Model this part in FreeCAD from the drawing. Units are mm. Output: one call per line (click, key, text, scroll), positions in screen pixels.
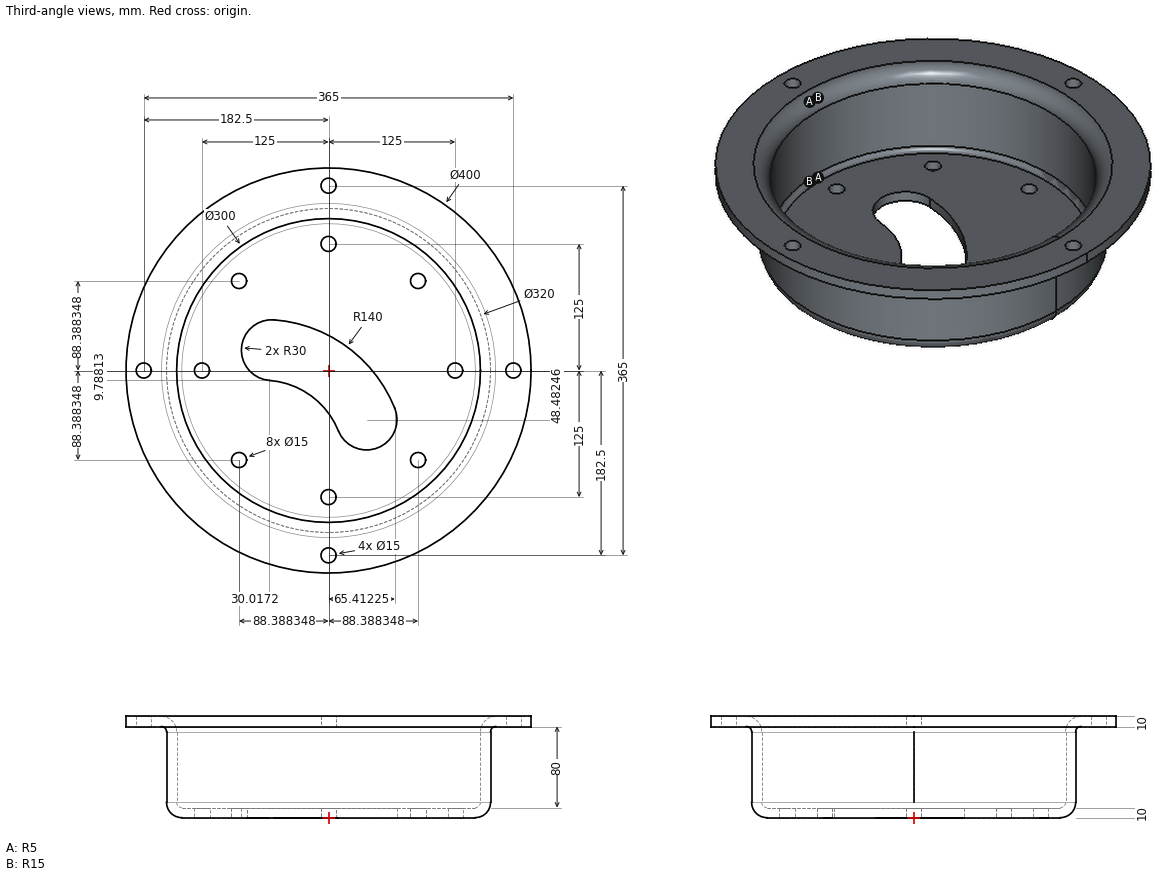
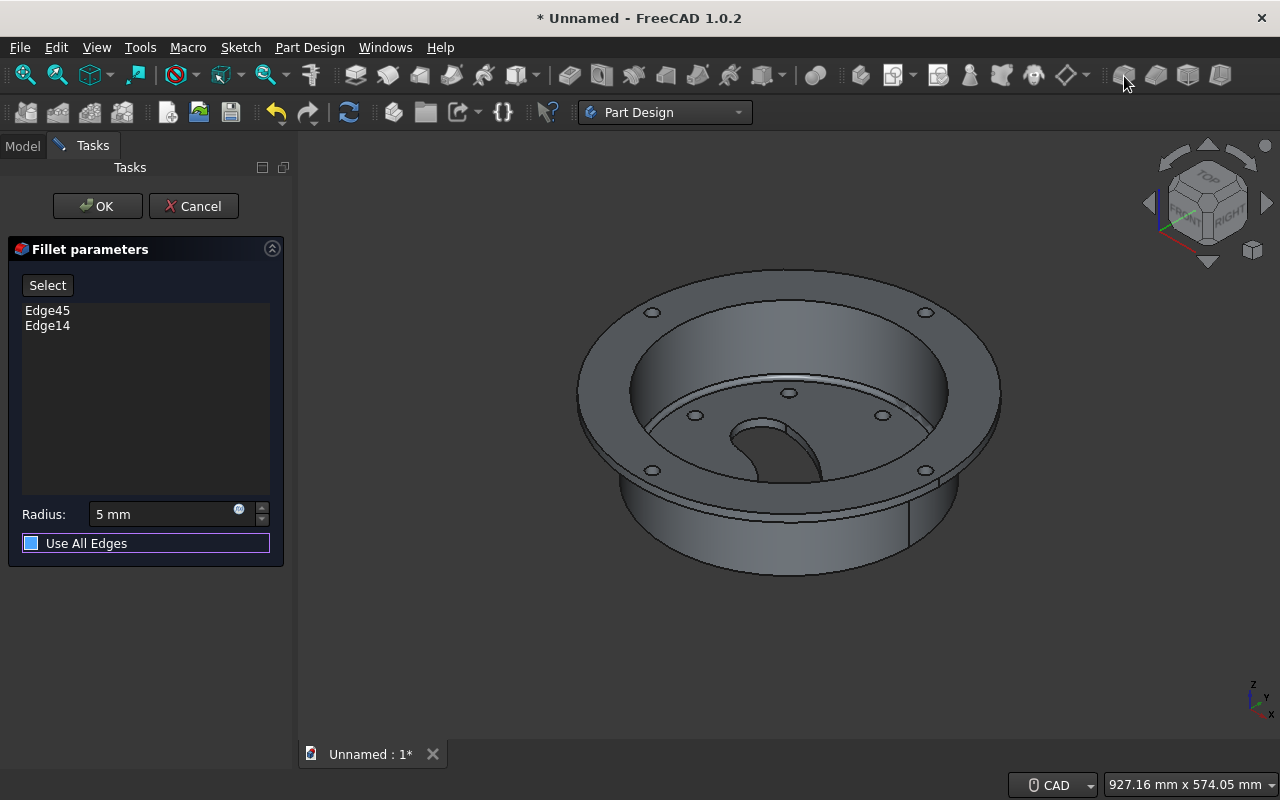
click(98, 206)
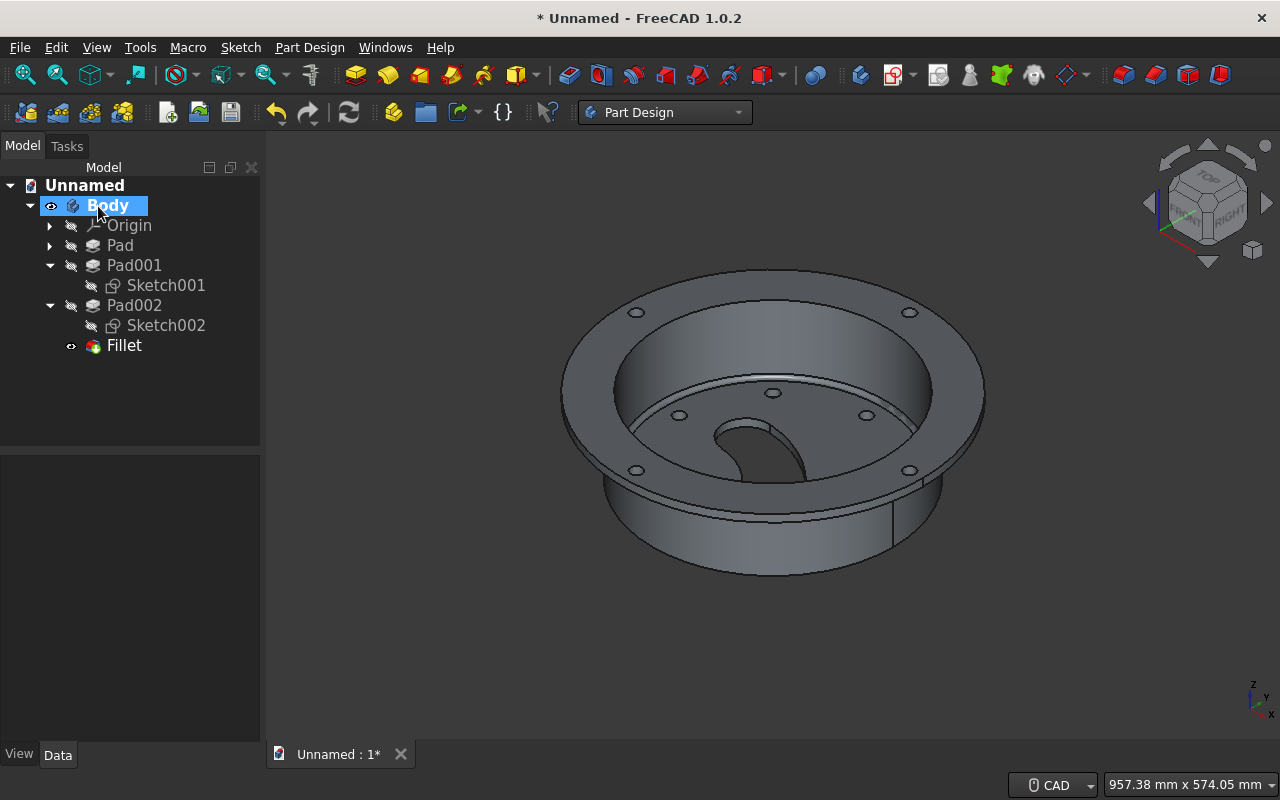
click(661, 326)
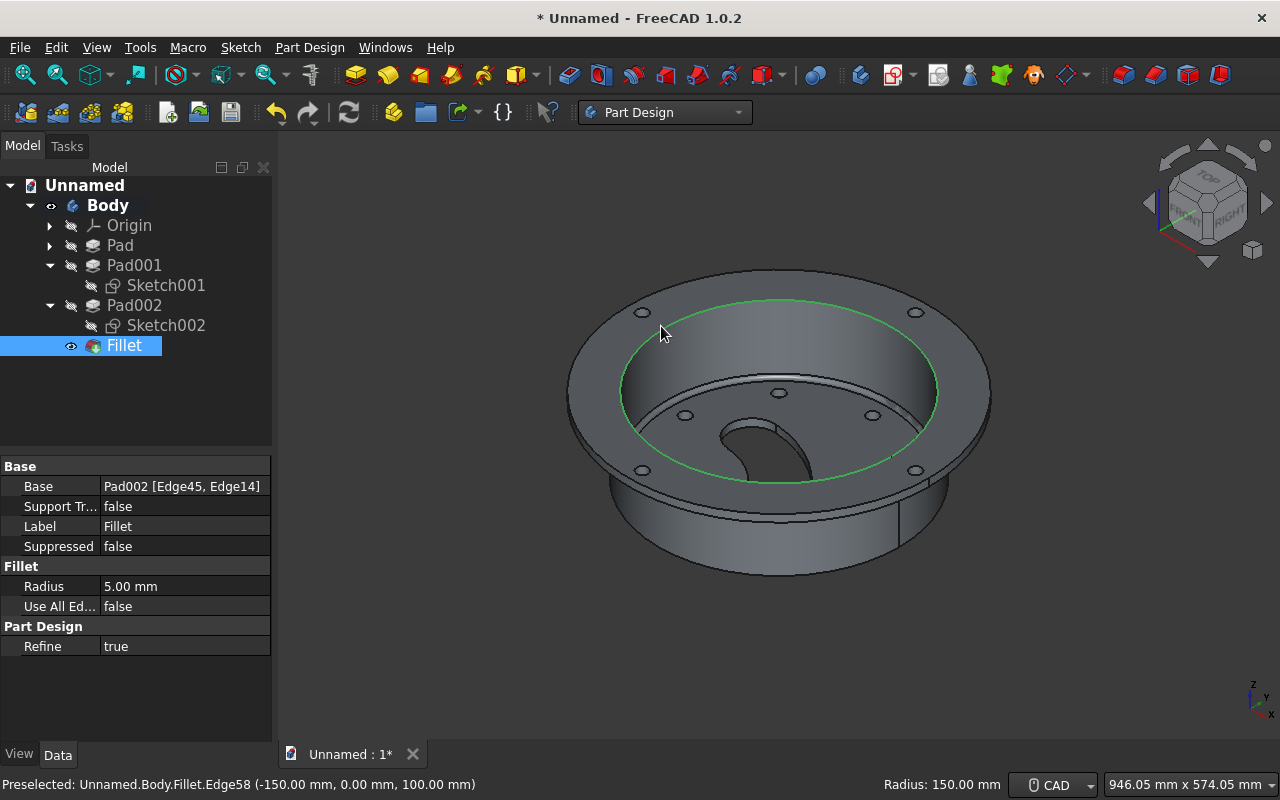
key(2)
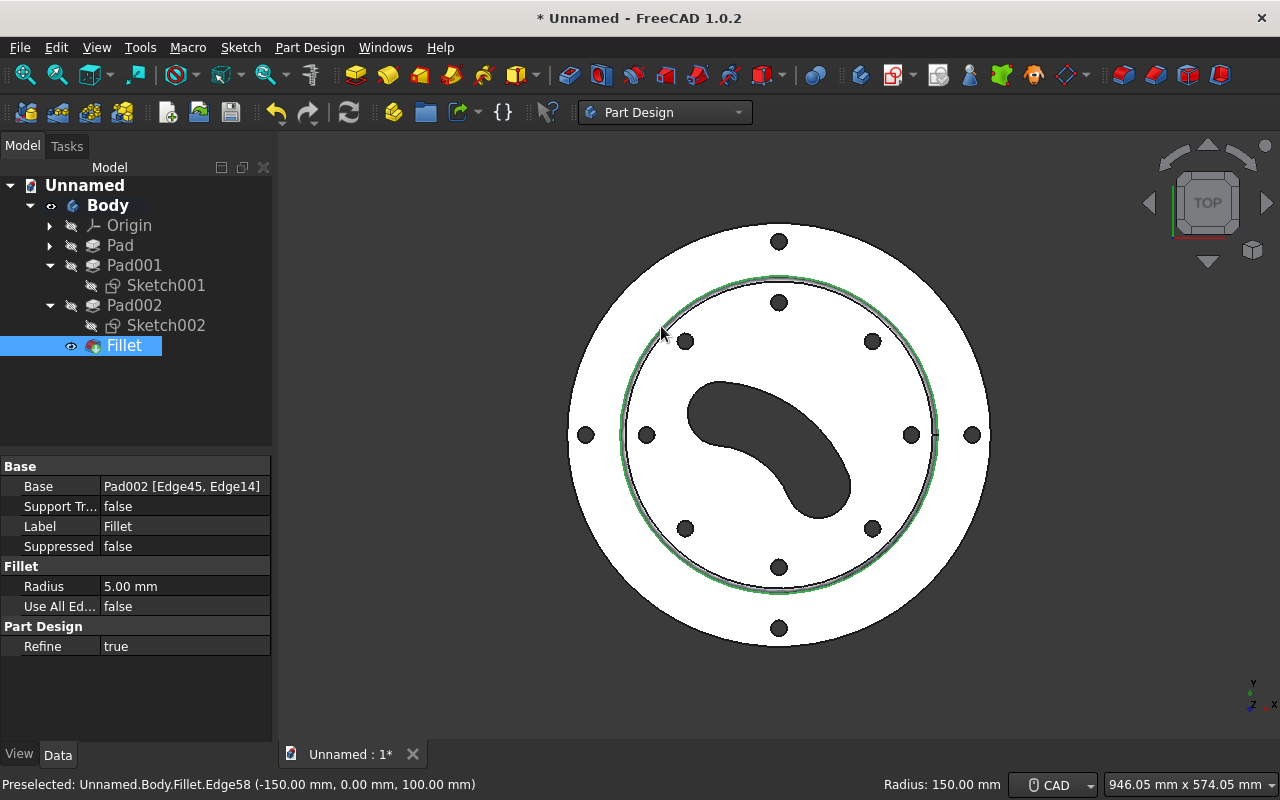
key(0)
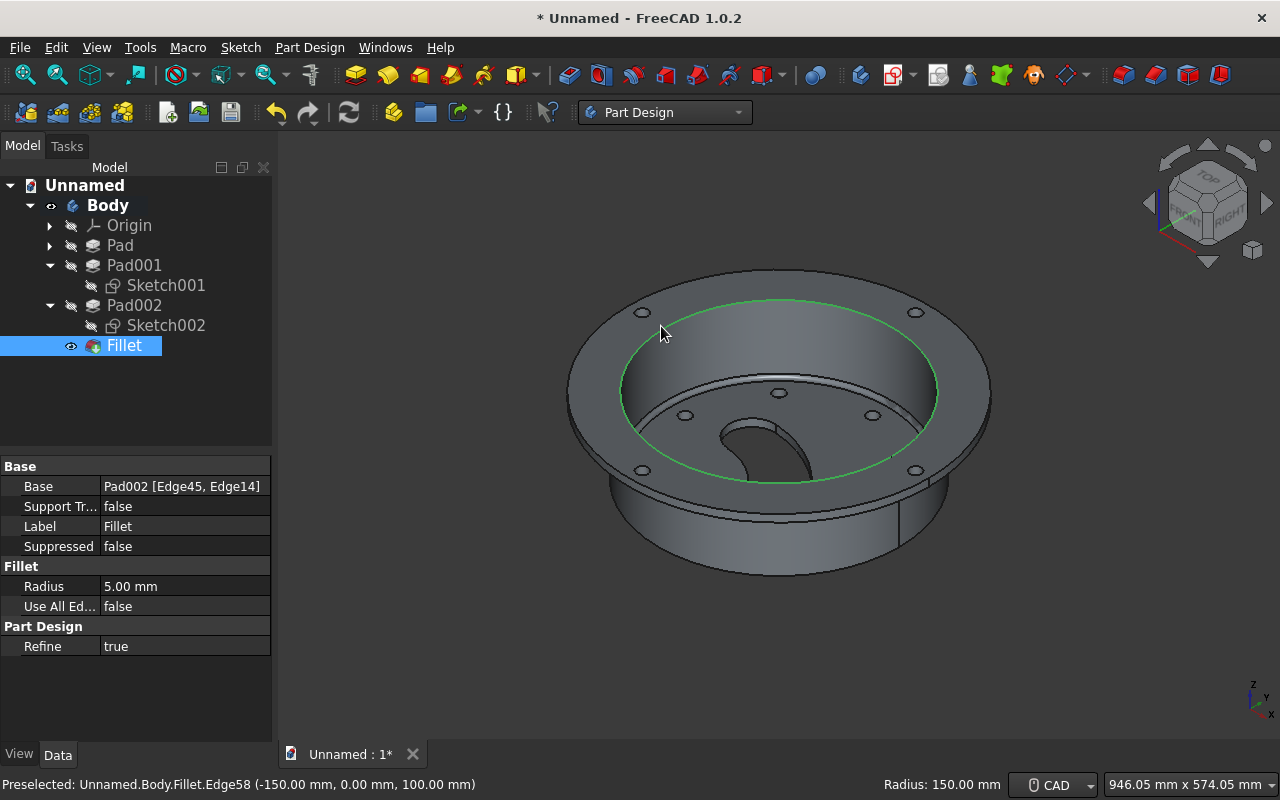
key(1)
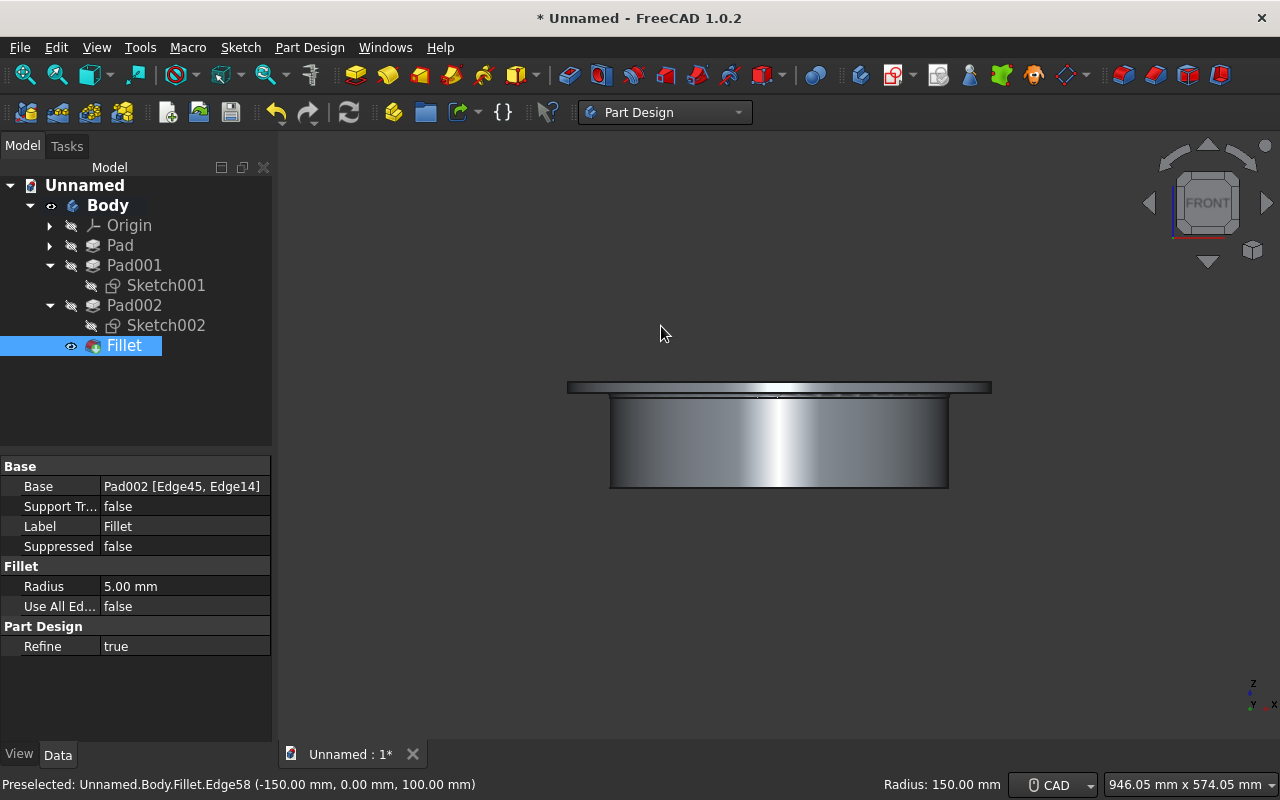
click(26, 76)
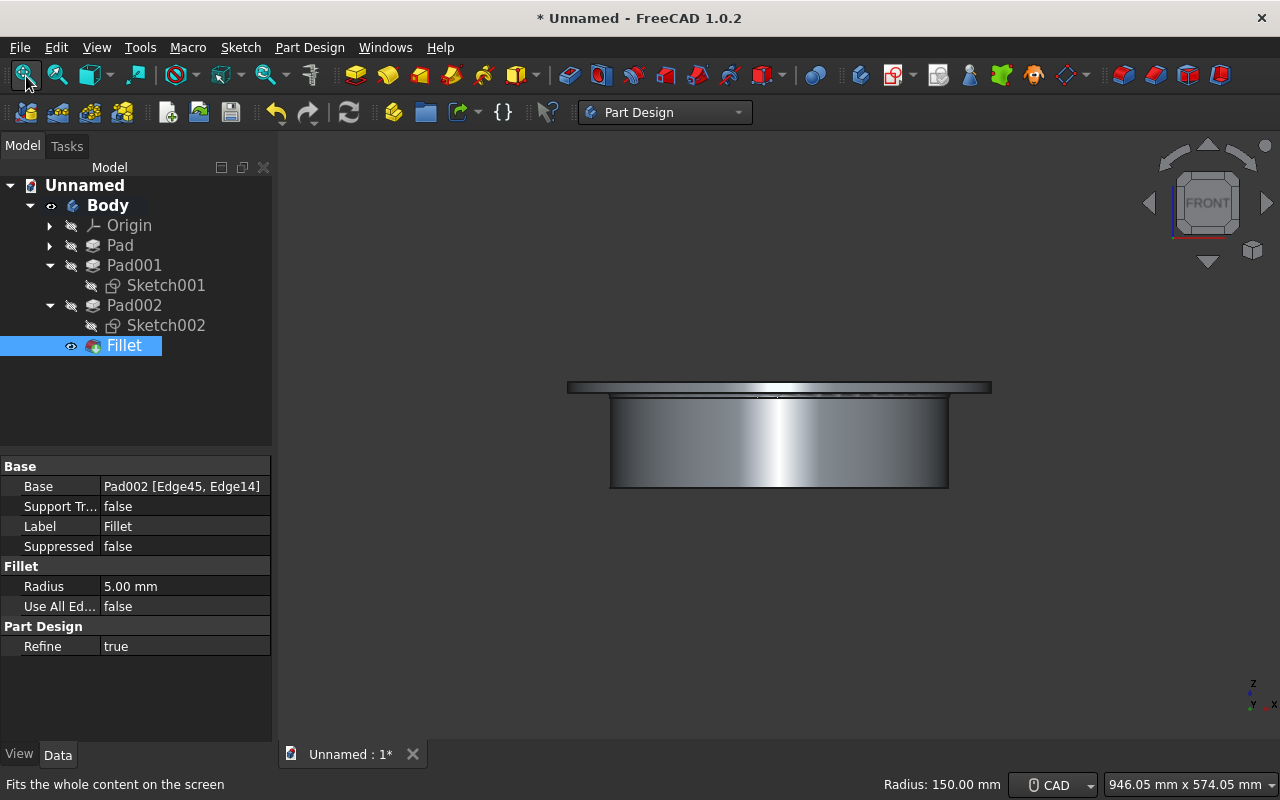
click(642, 487, ctrl)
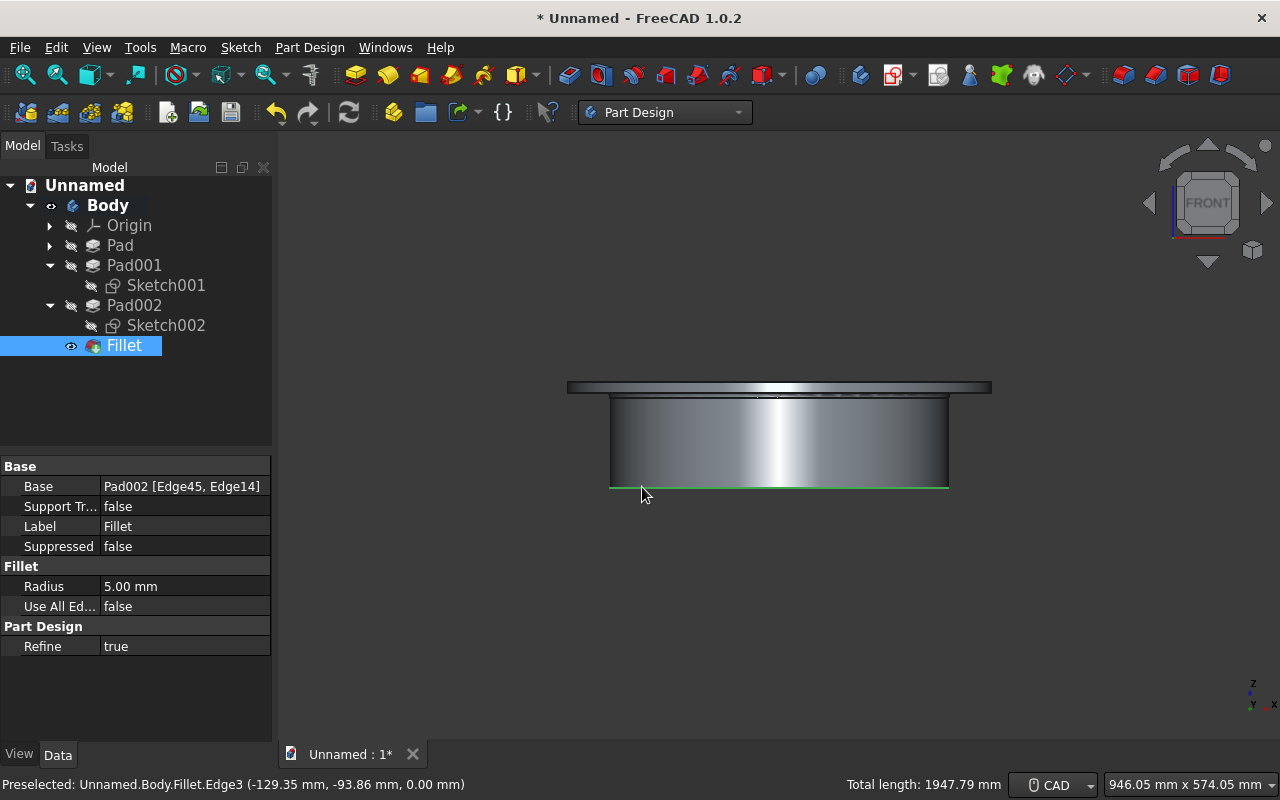
click(1124, 76)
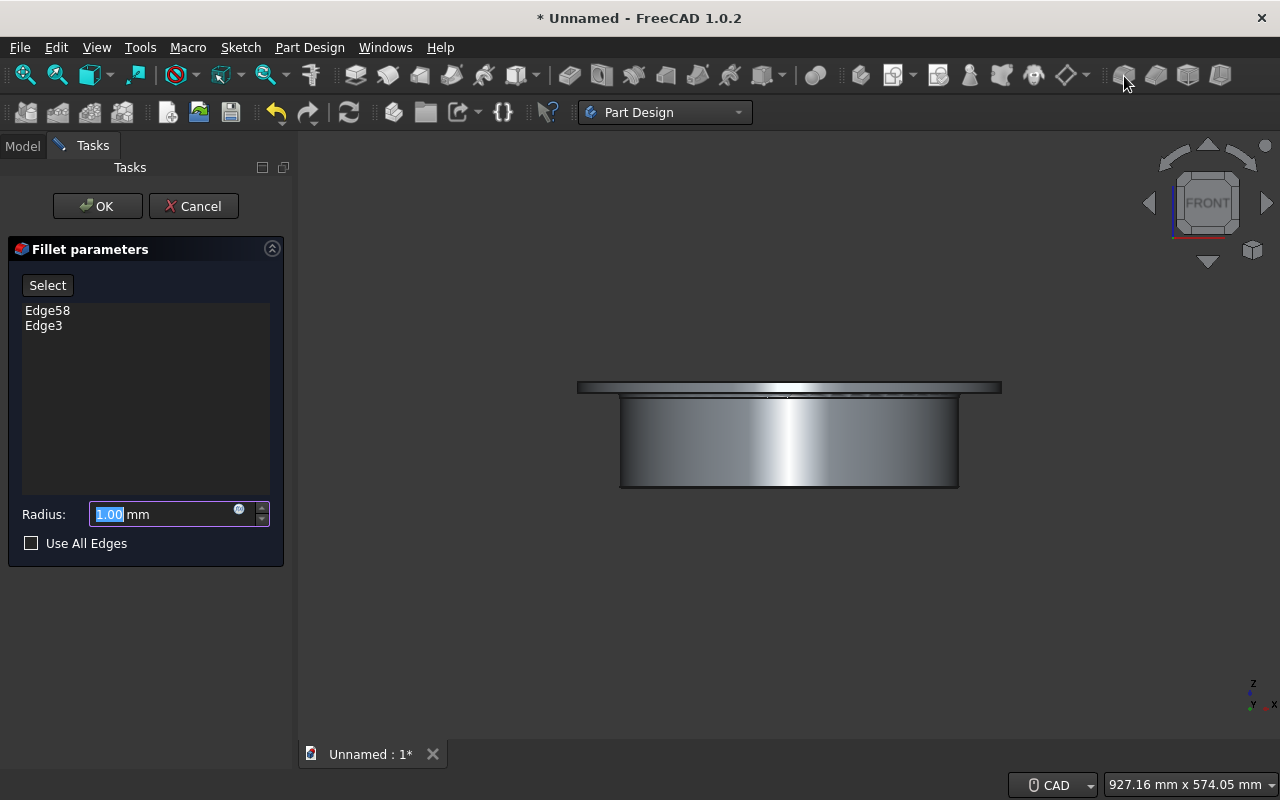
text(15)
key(Tab)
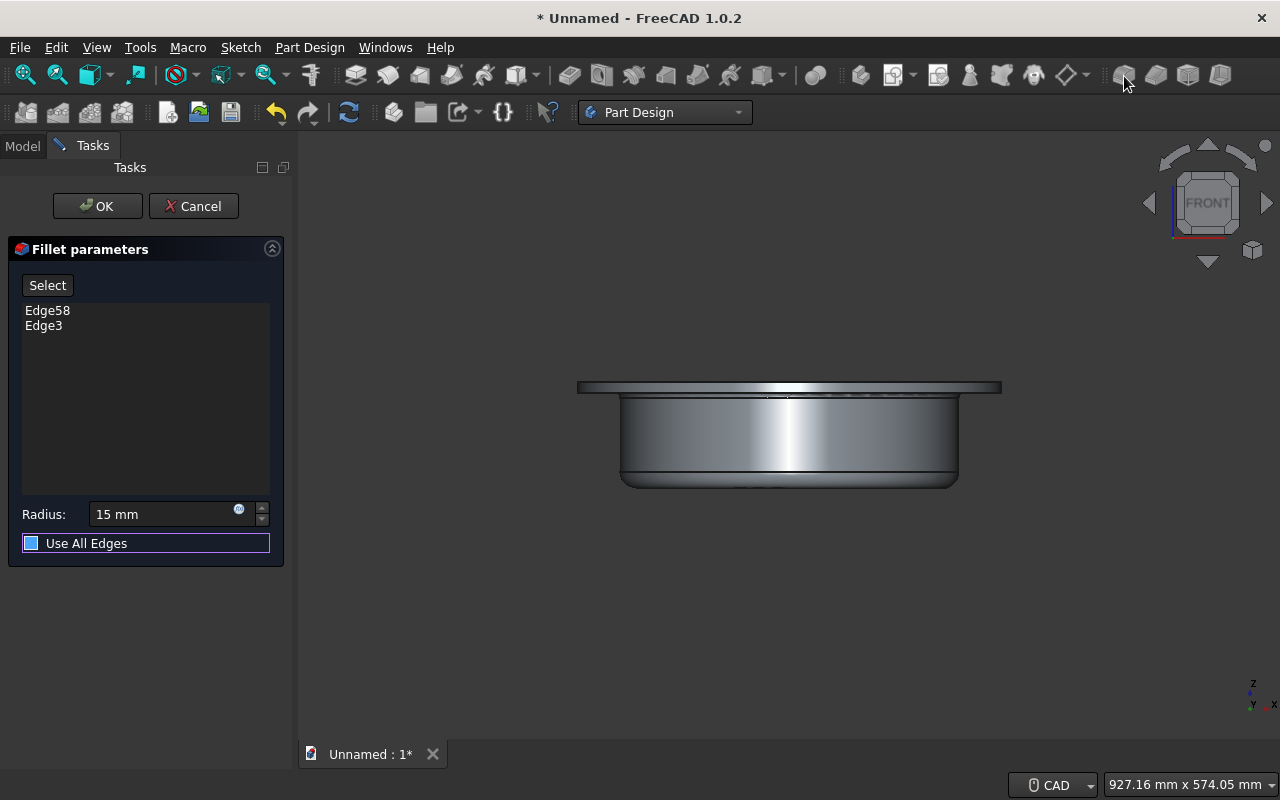
click(98, 206)